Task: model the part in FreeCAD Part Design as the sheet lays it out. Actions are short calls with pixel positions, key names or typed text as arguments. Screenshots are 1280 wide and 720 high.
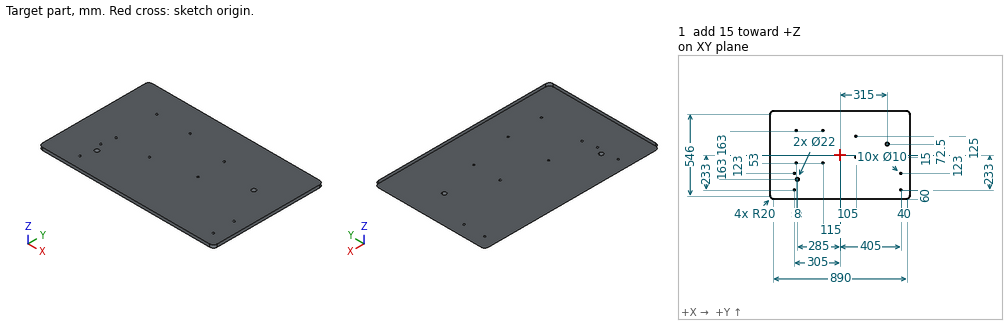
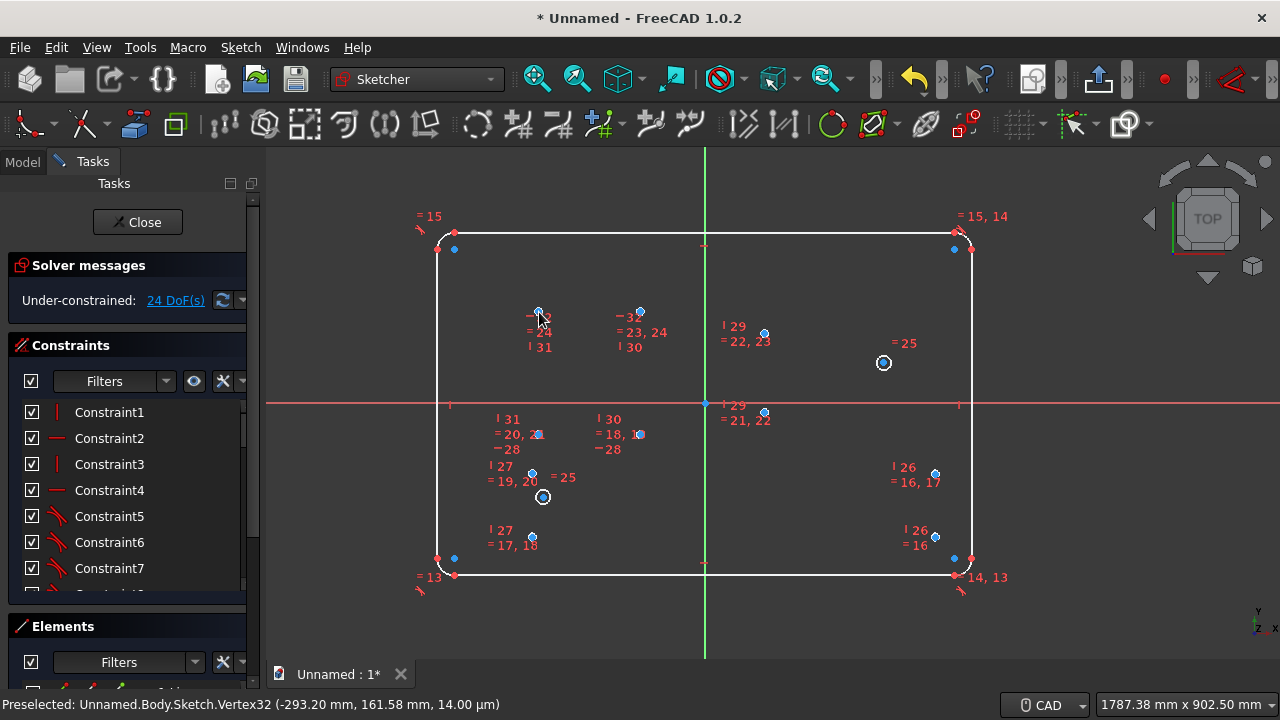
click(1232, 80)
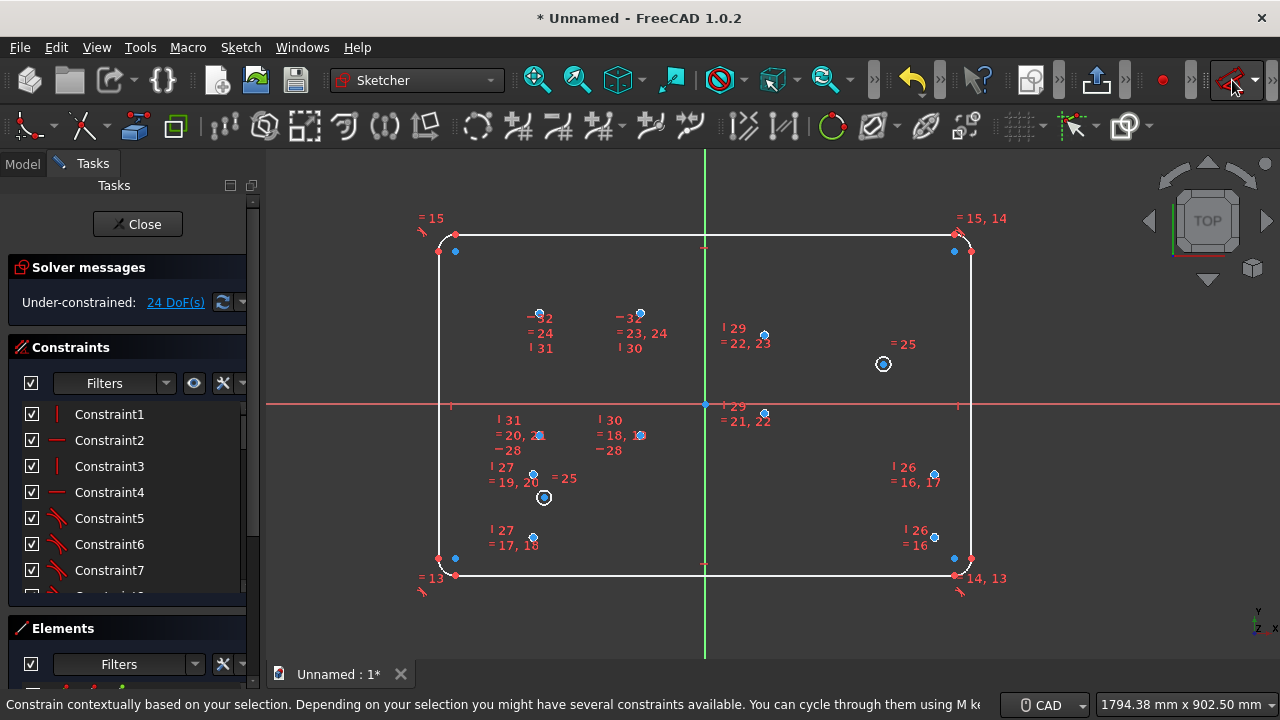
scroll(444, 571, up, 7)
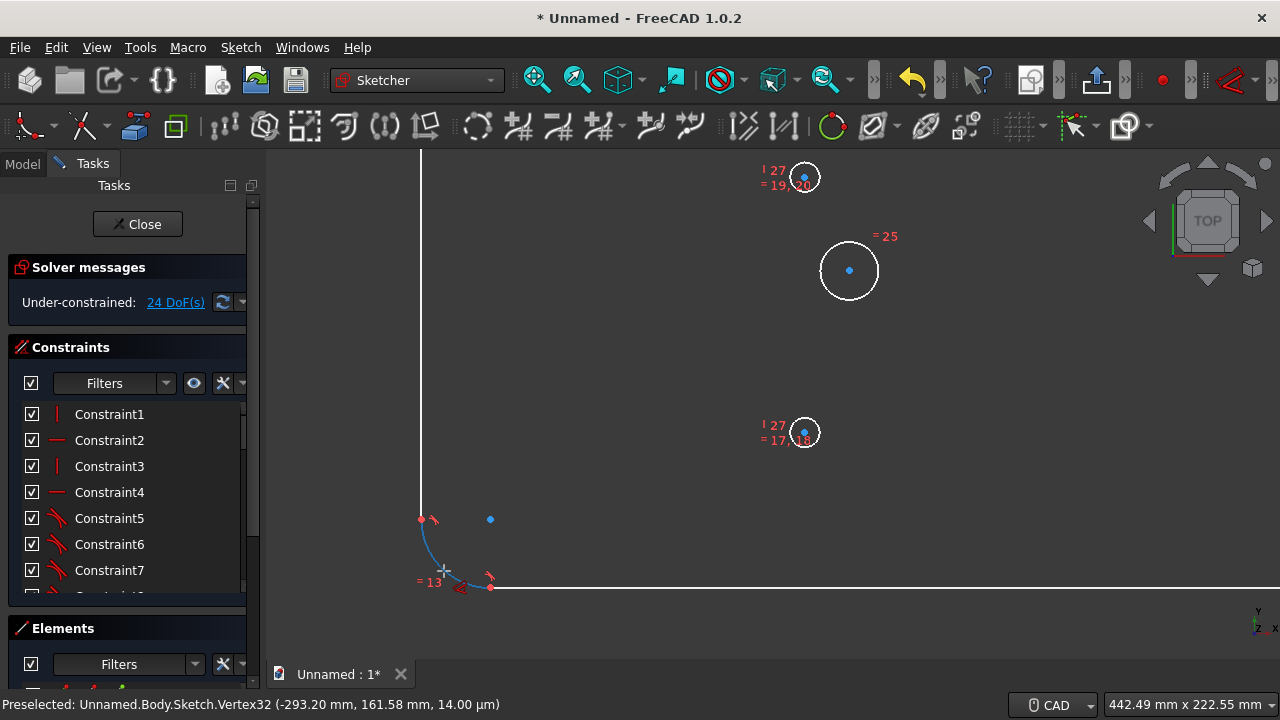
click(442, 568)
click(420, 591)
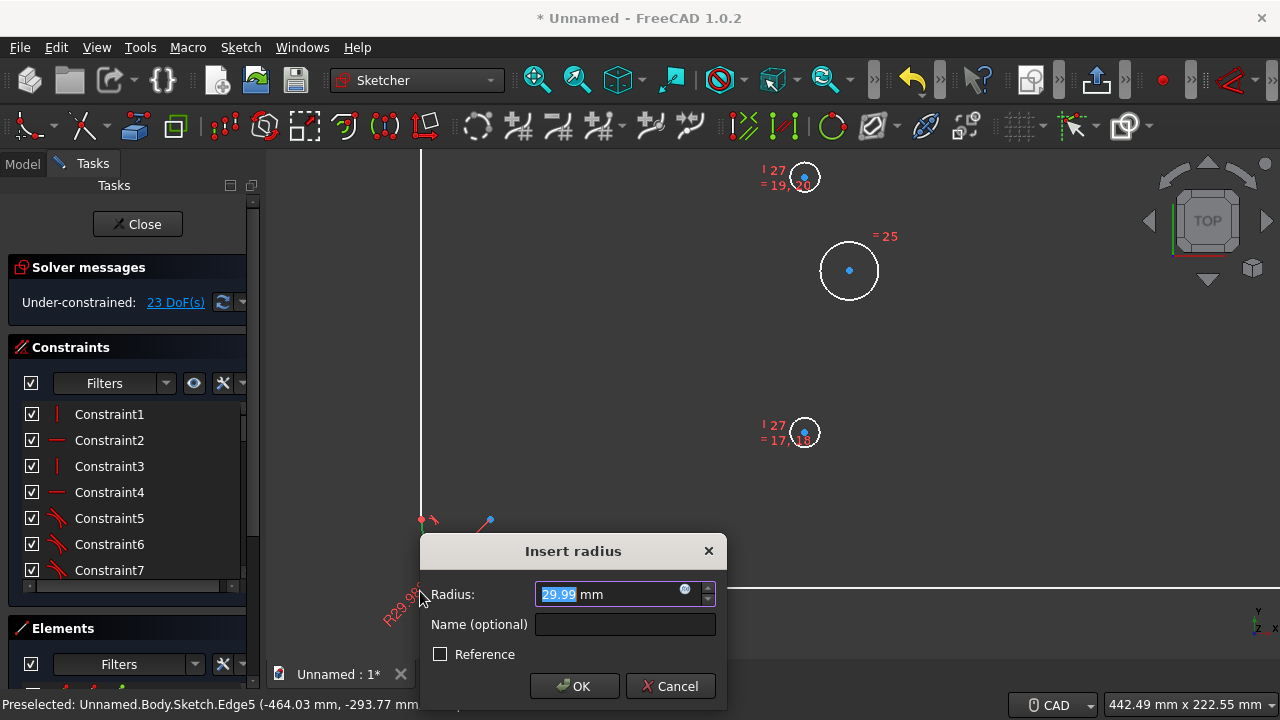
text(20)
key(Return)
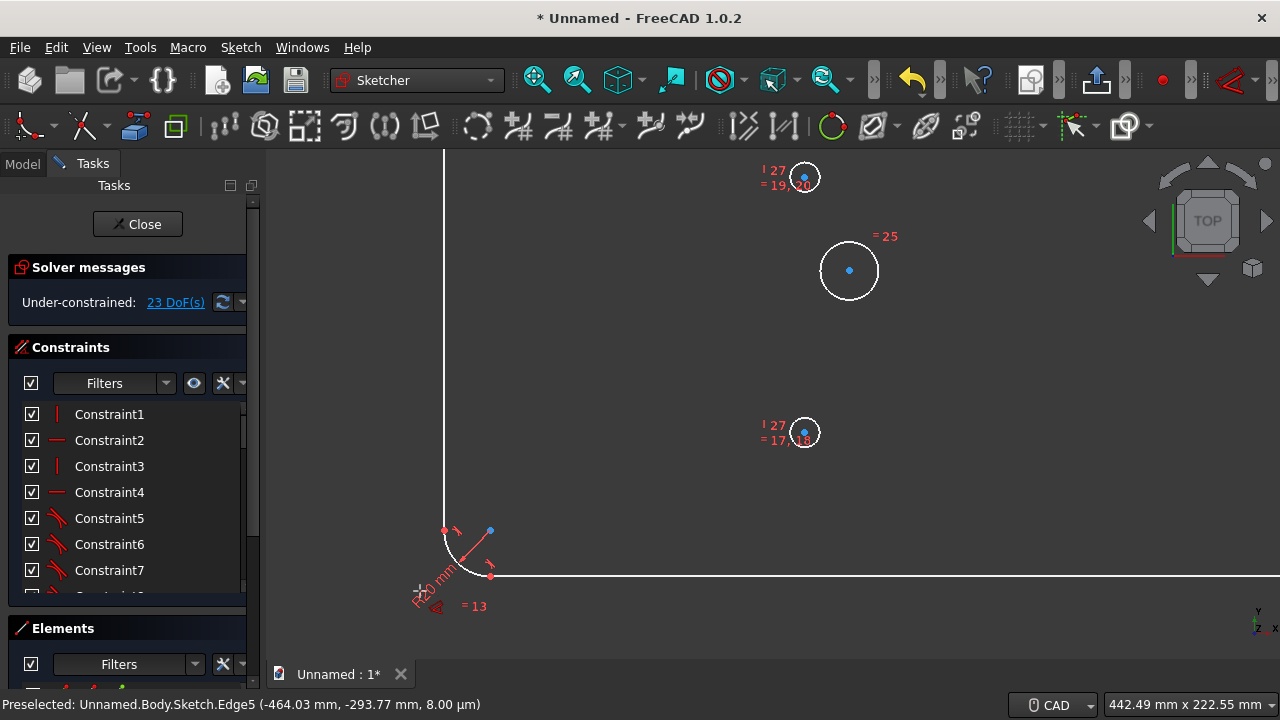
scroll(443, 571, down, 7)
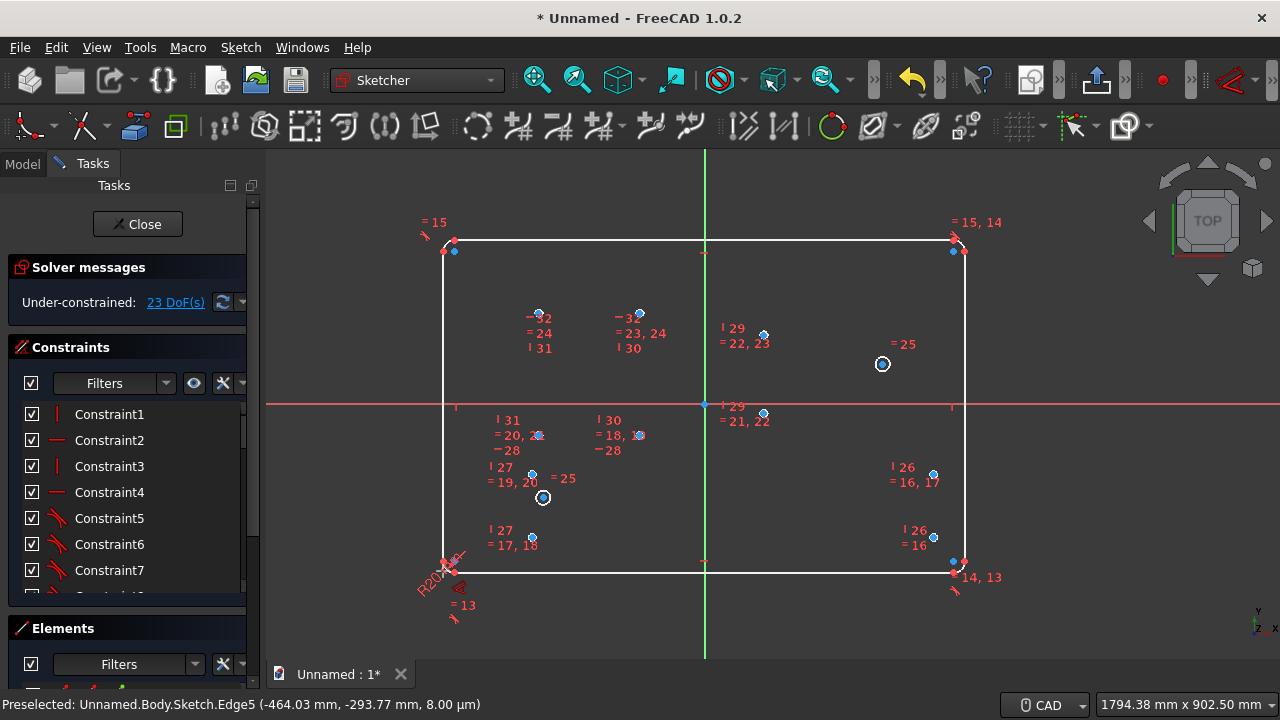
scroll(936, 535, up, 10)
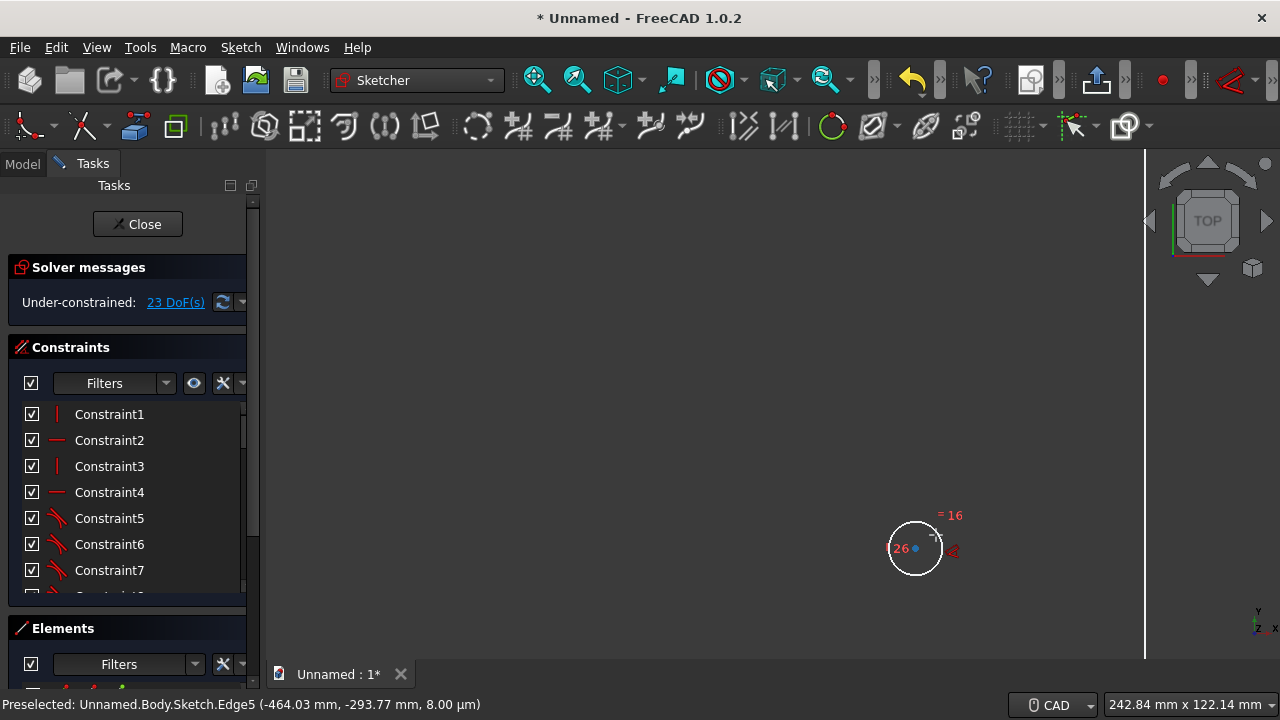
click(934, 530)
click(957, 507)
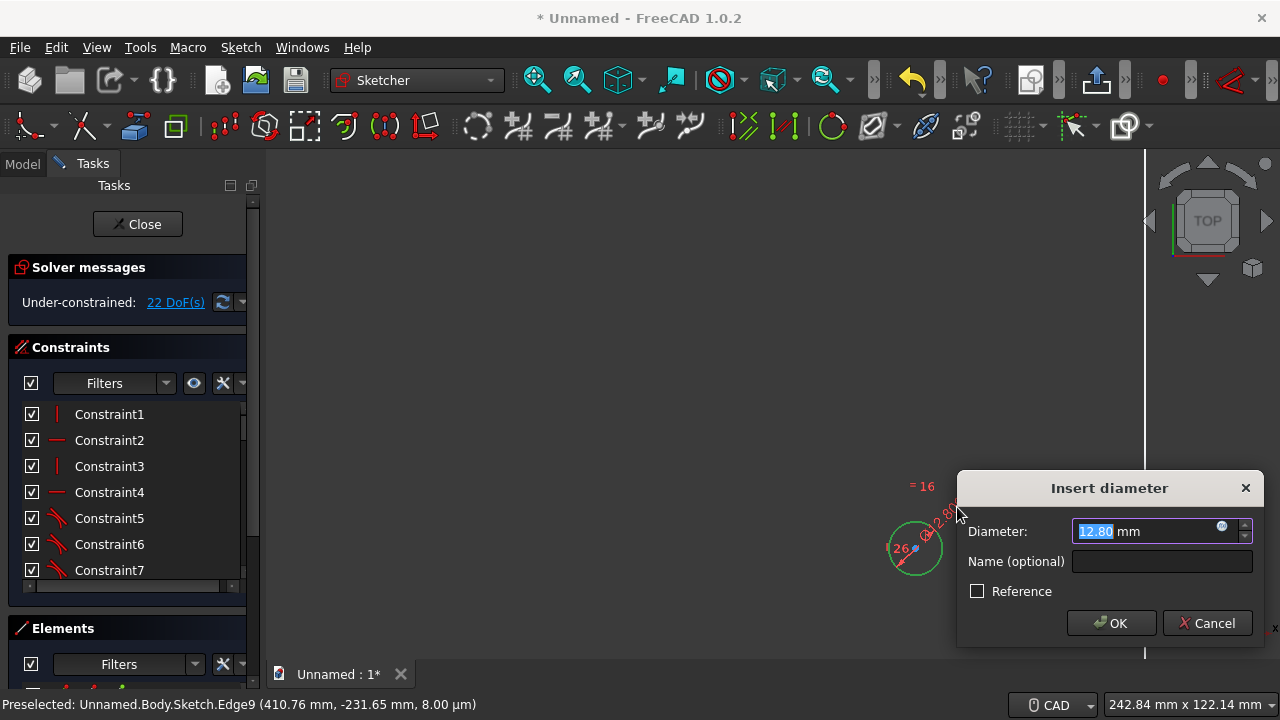
text(10)
key(Return)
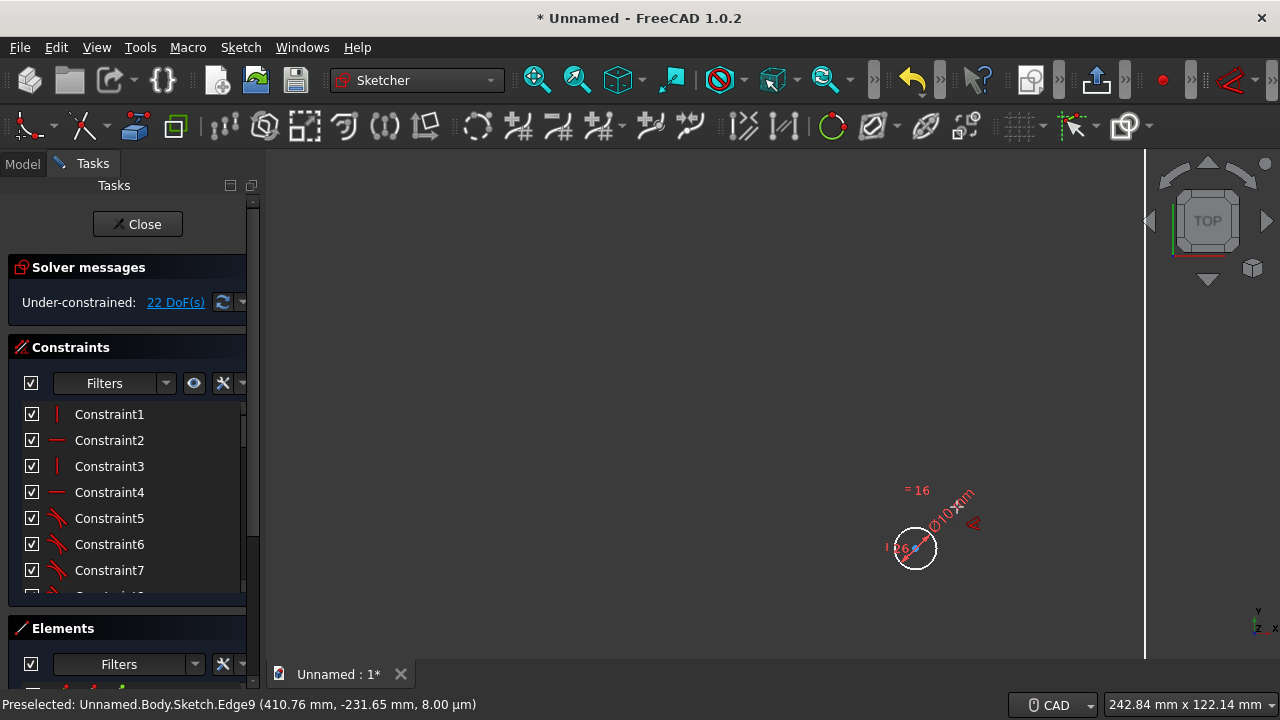
scroll(937, 535, down, 10)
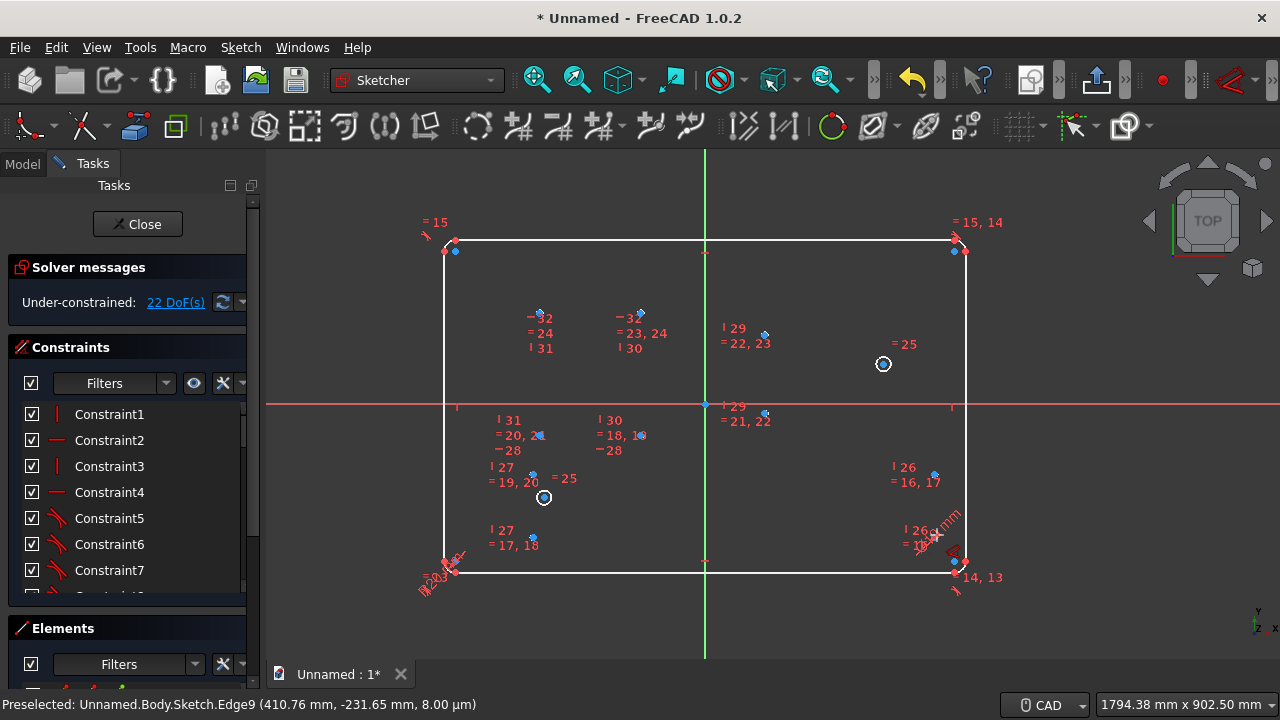
scroll(549, 493, up, 6)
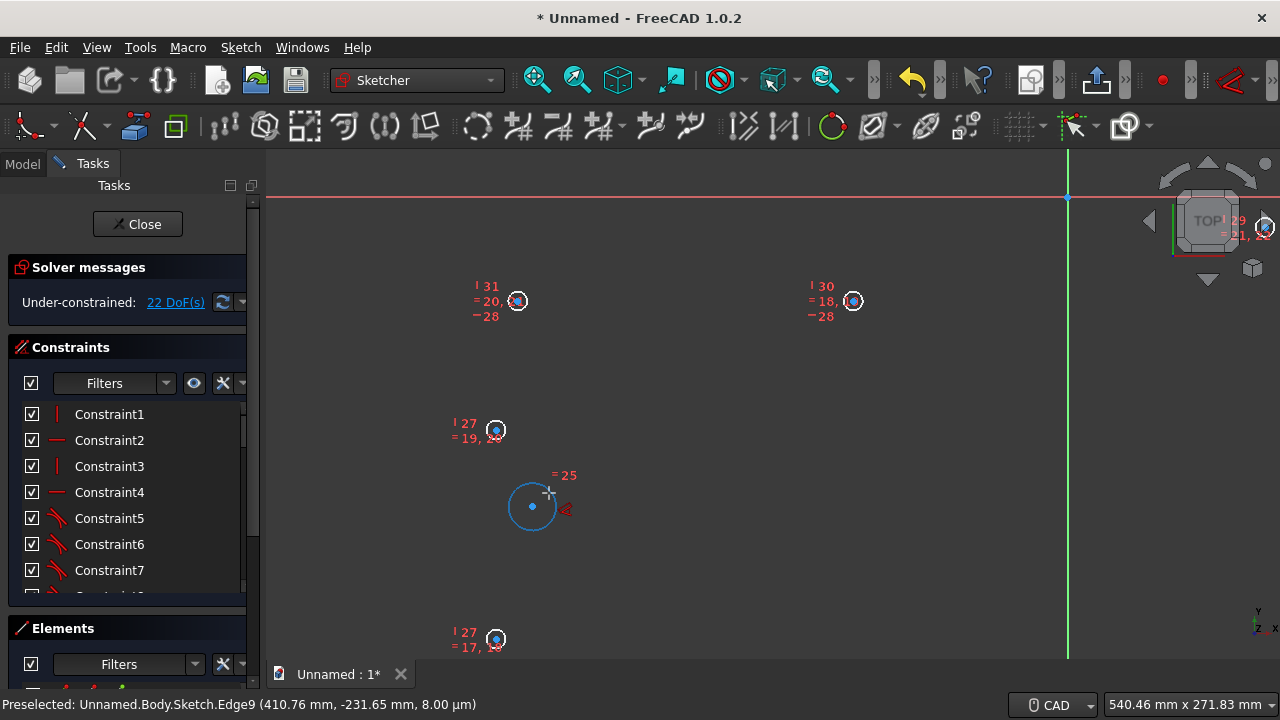
click(549, 490)
click(571, 467)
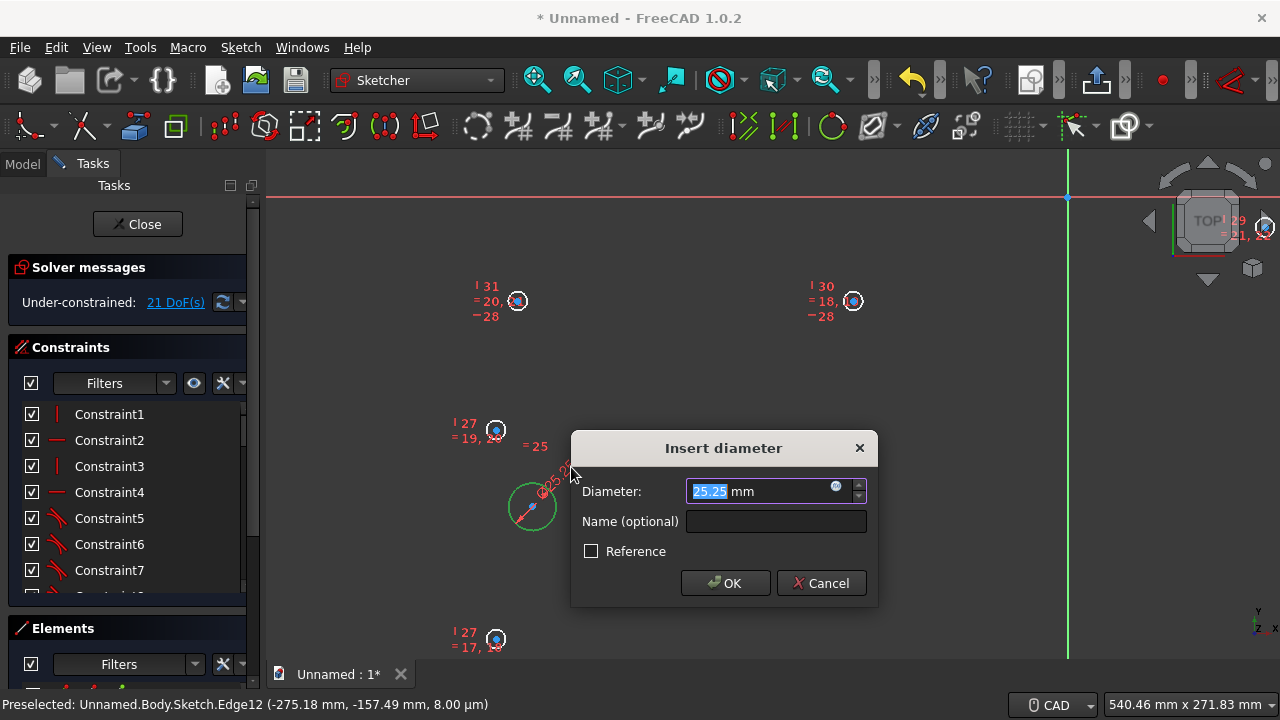
text(22)
key(Return)